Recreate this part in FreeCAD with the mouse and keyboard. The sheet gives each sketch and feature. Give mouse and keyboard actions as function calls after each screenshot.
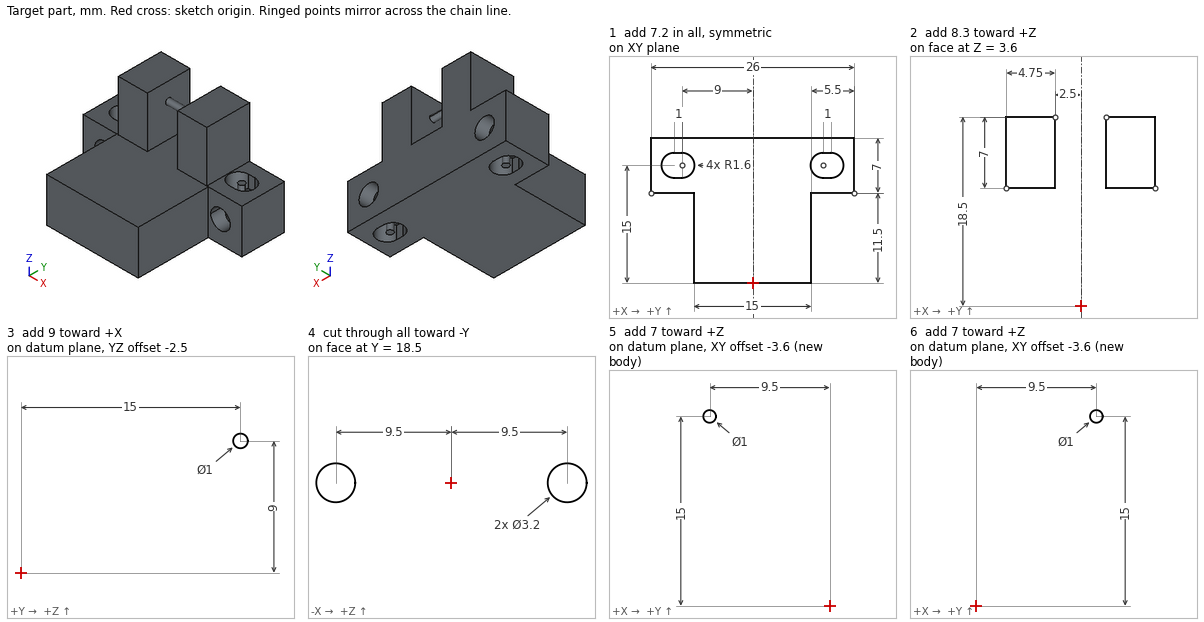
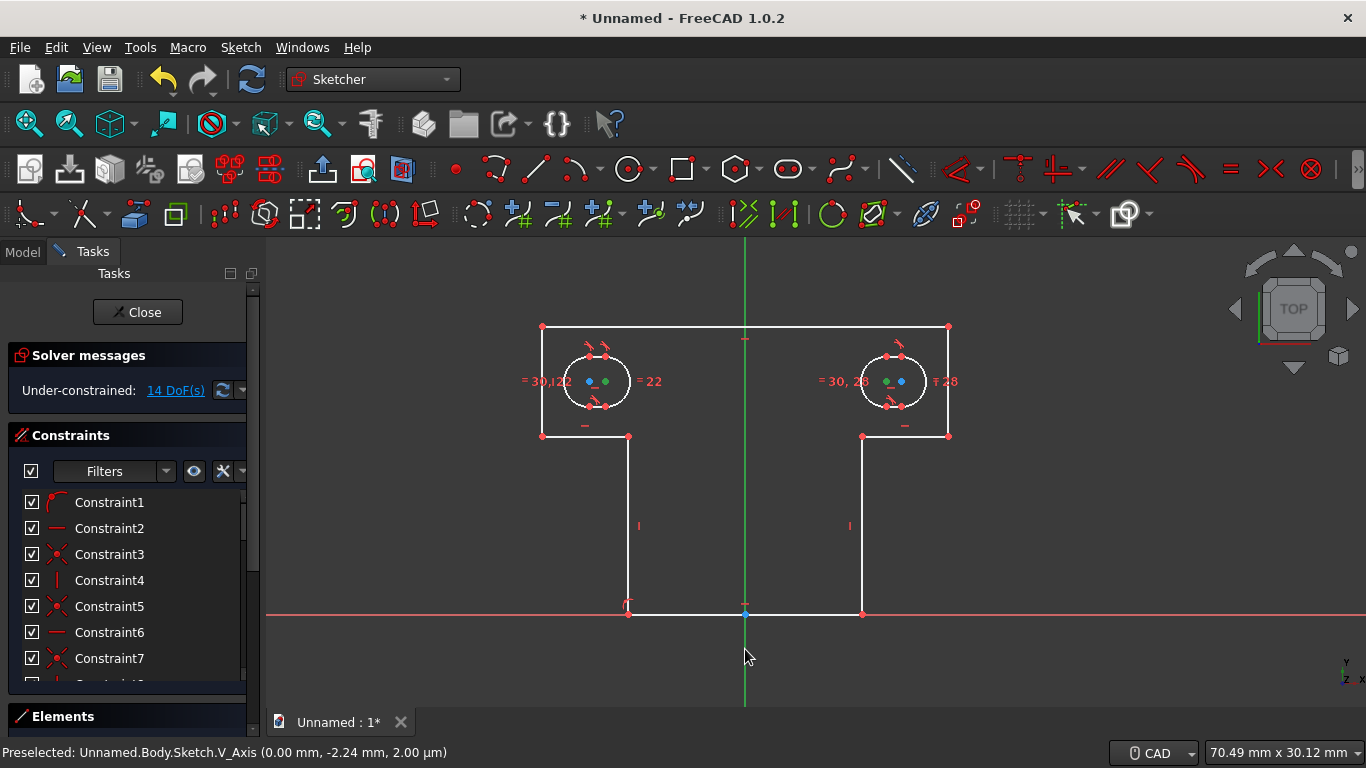
click(1272, 170)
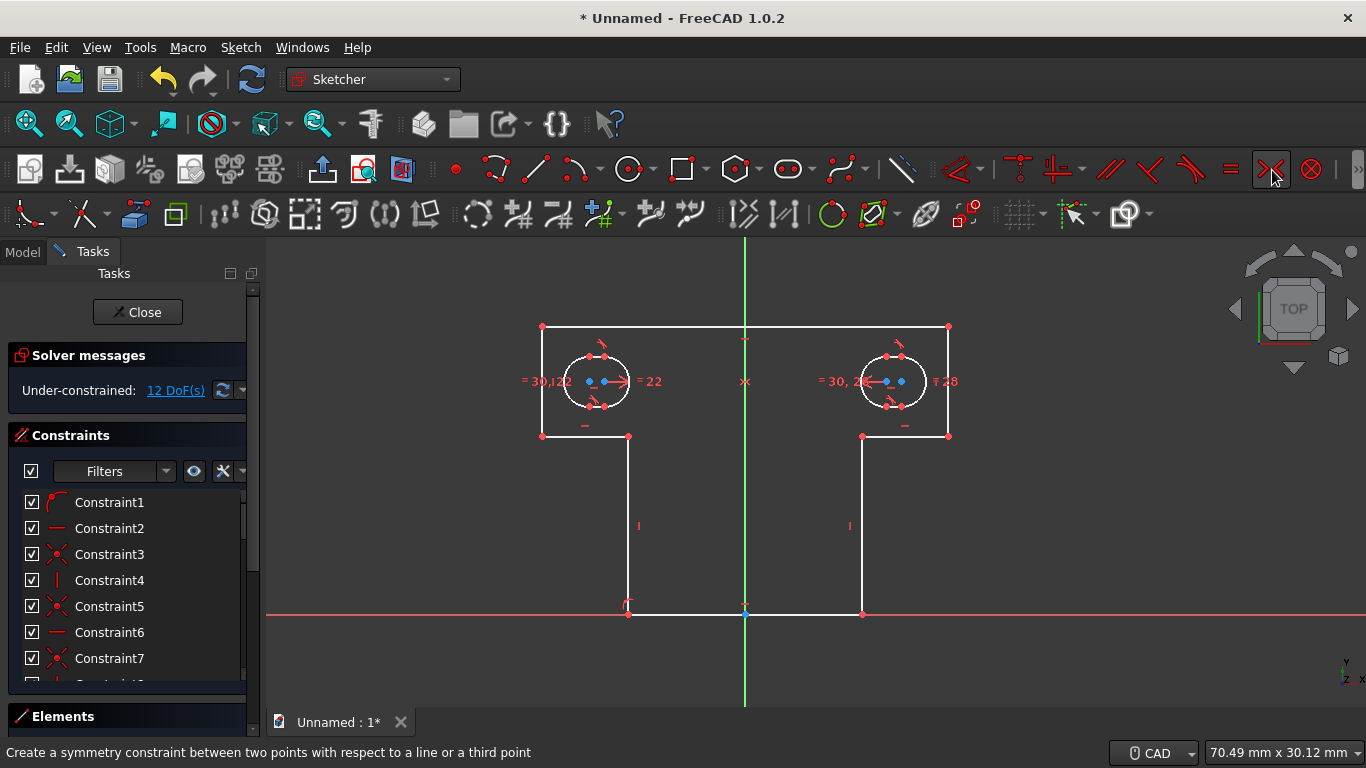
click(948, 437)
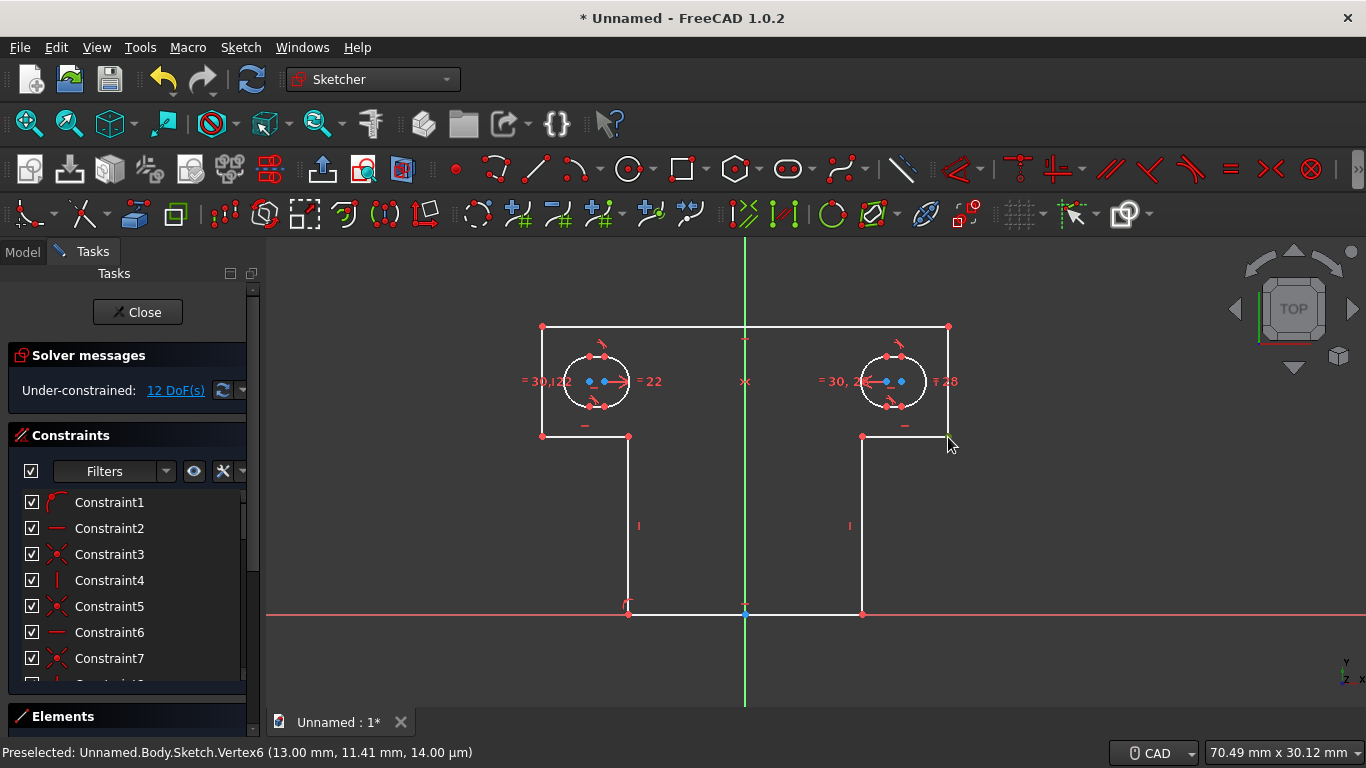
click(542, 437)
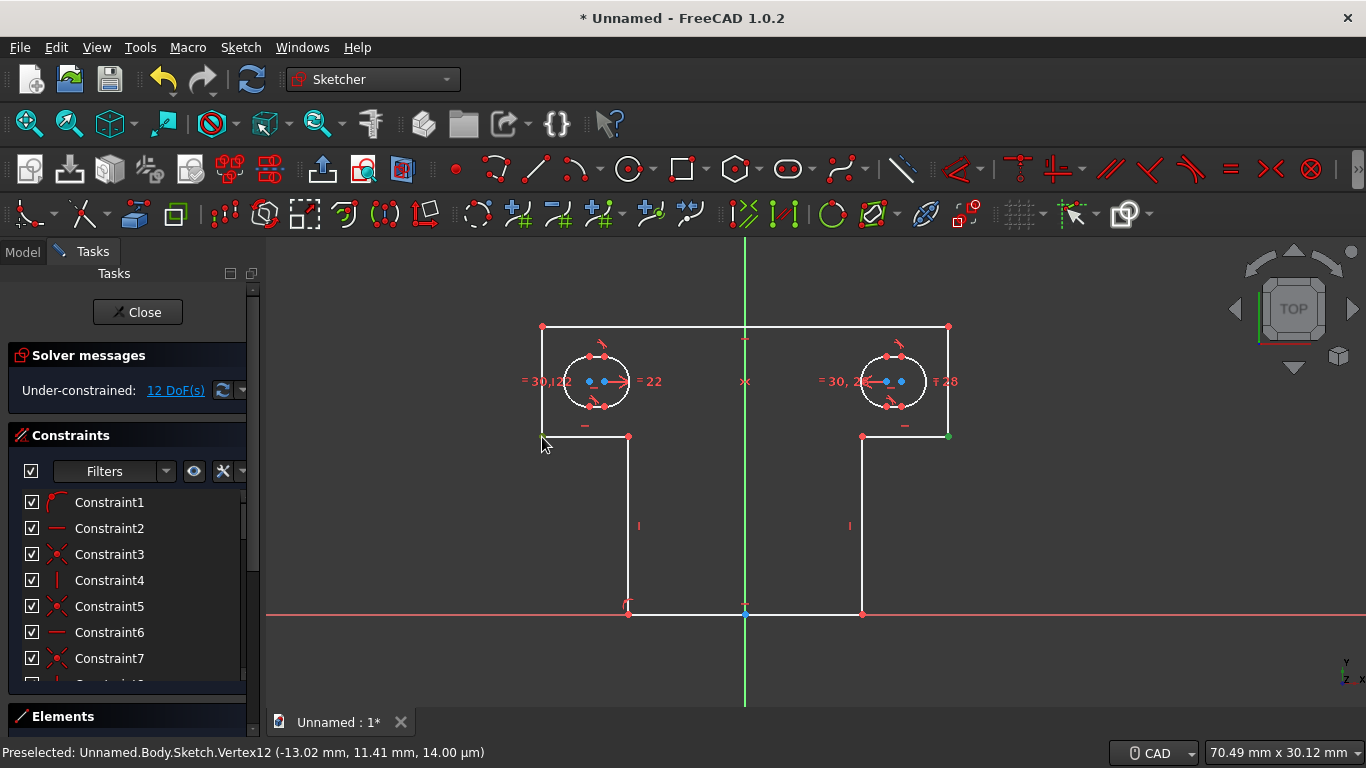
click(745, 649)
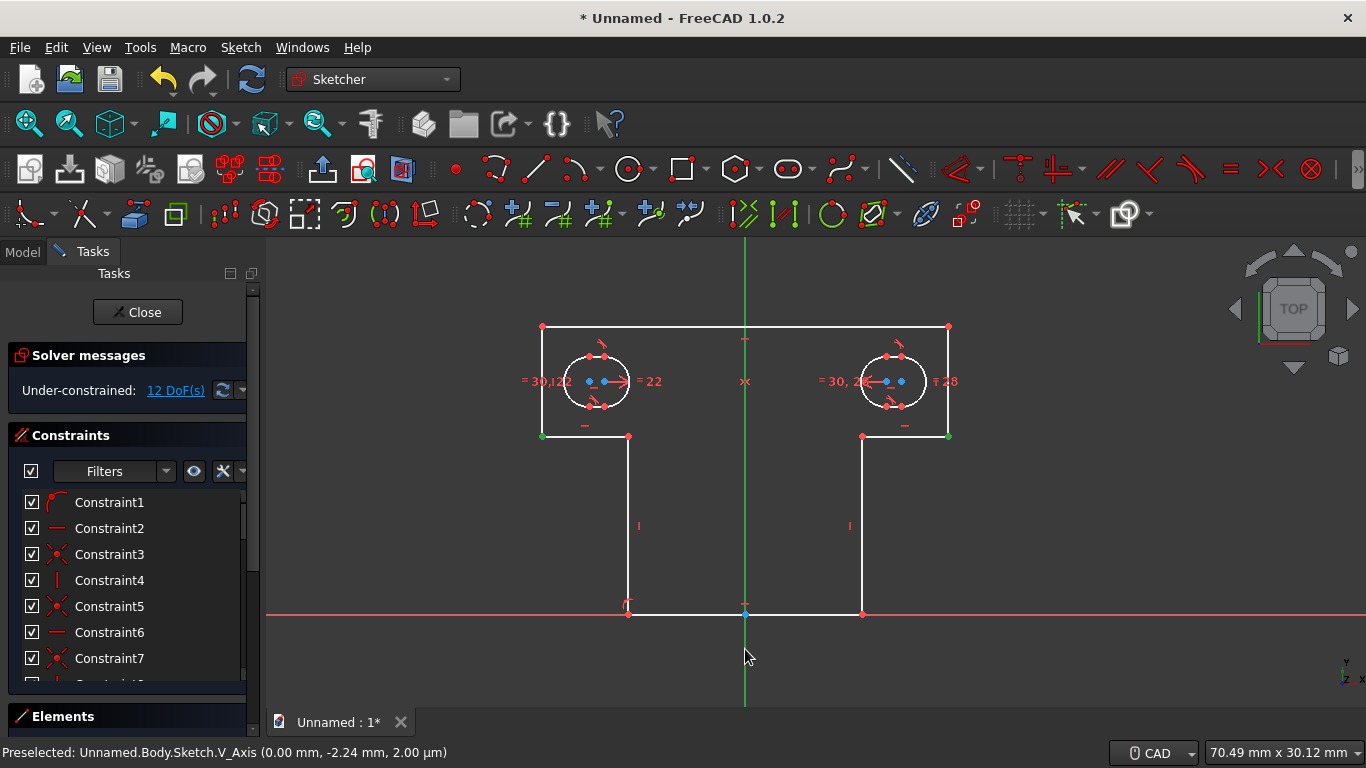
key(s)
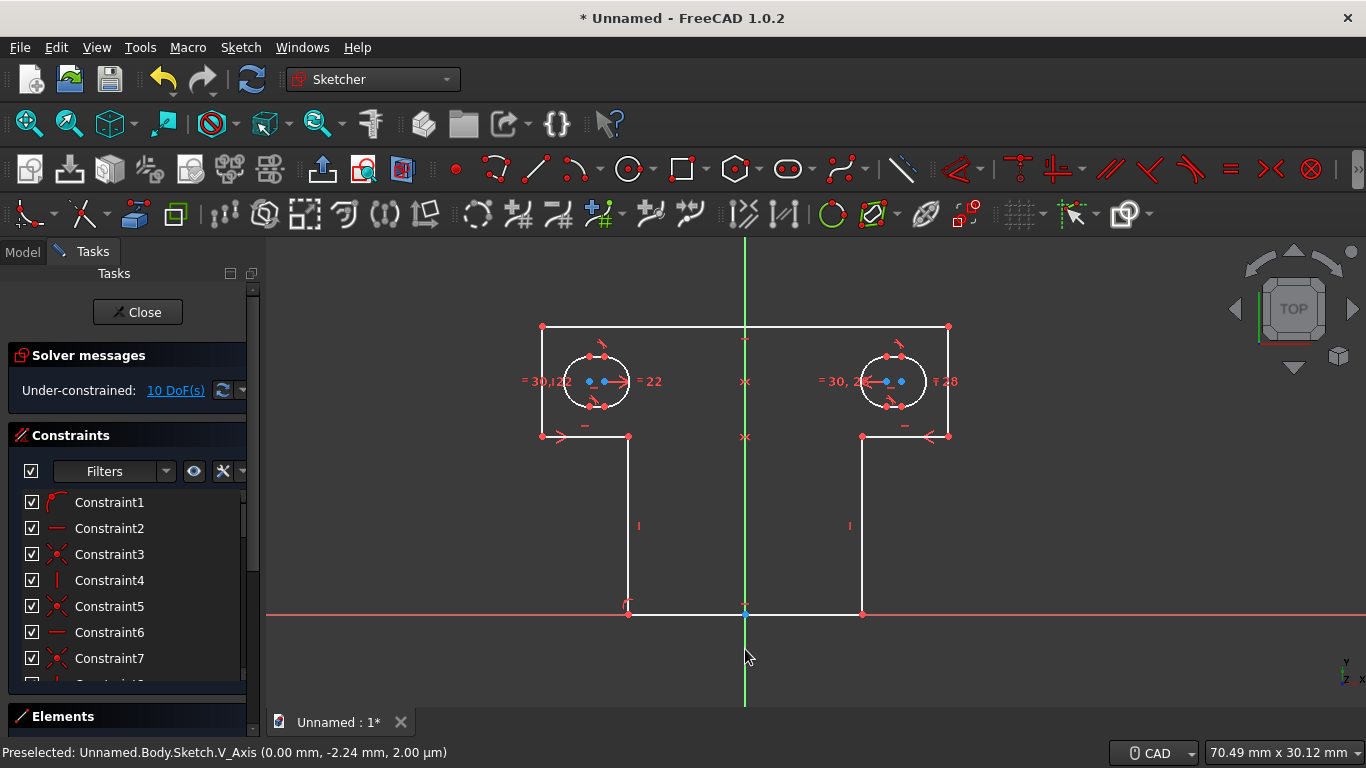
scroll(569, 367, up, 3)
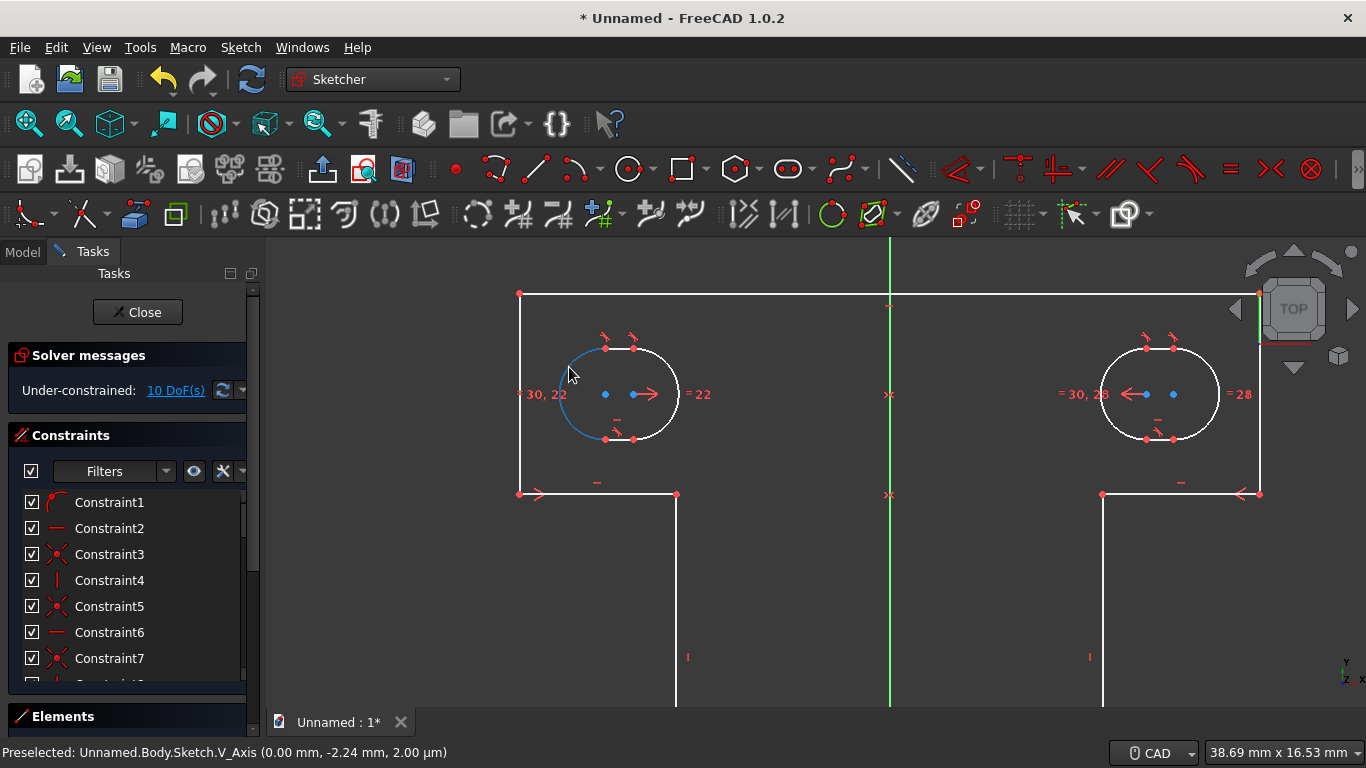
click(568, 367)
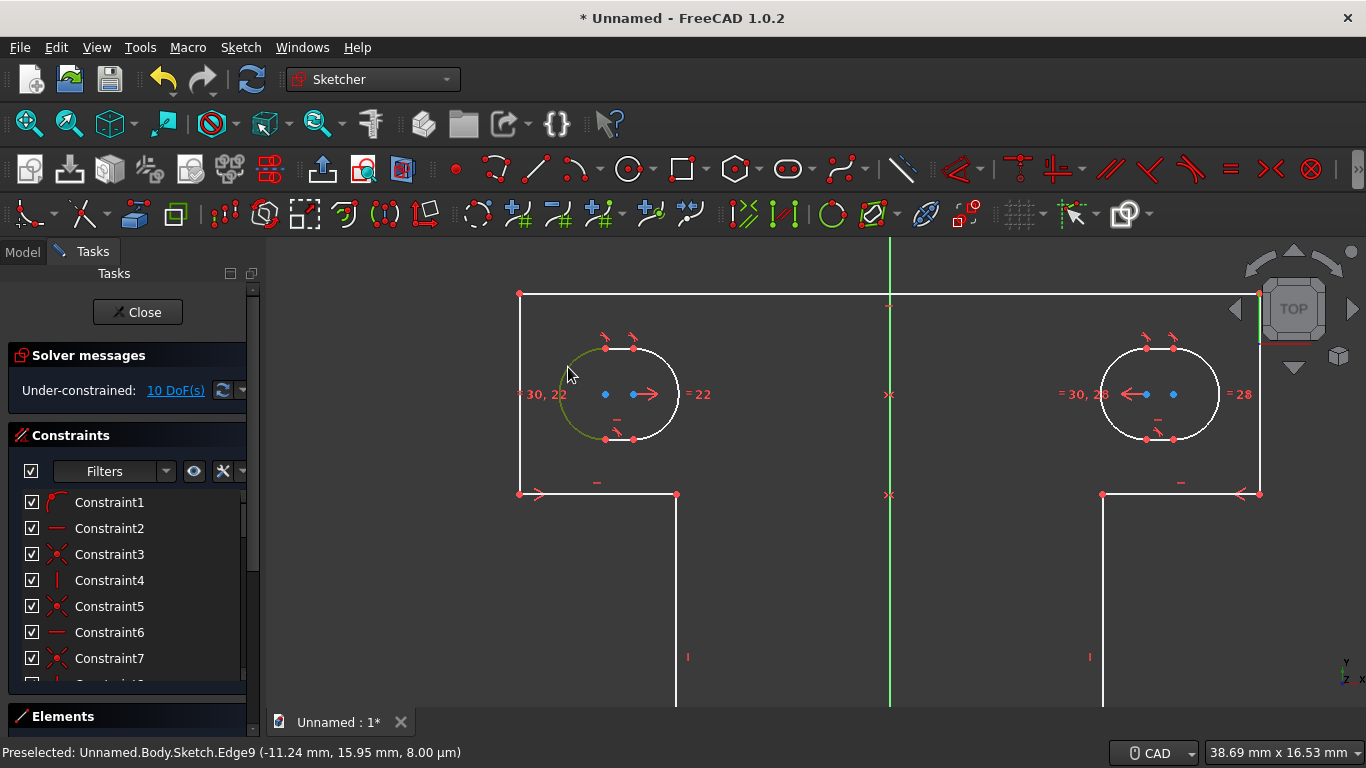
key(k)
key(r)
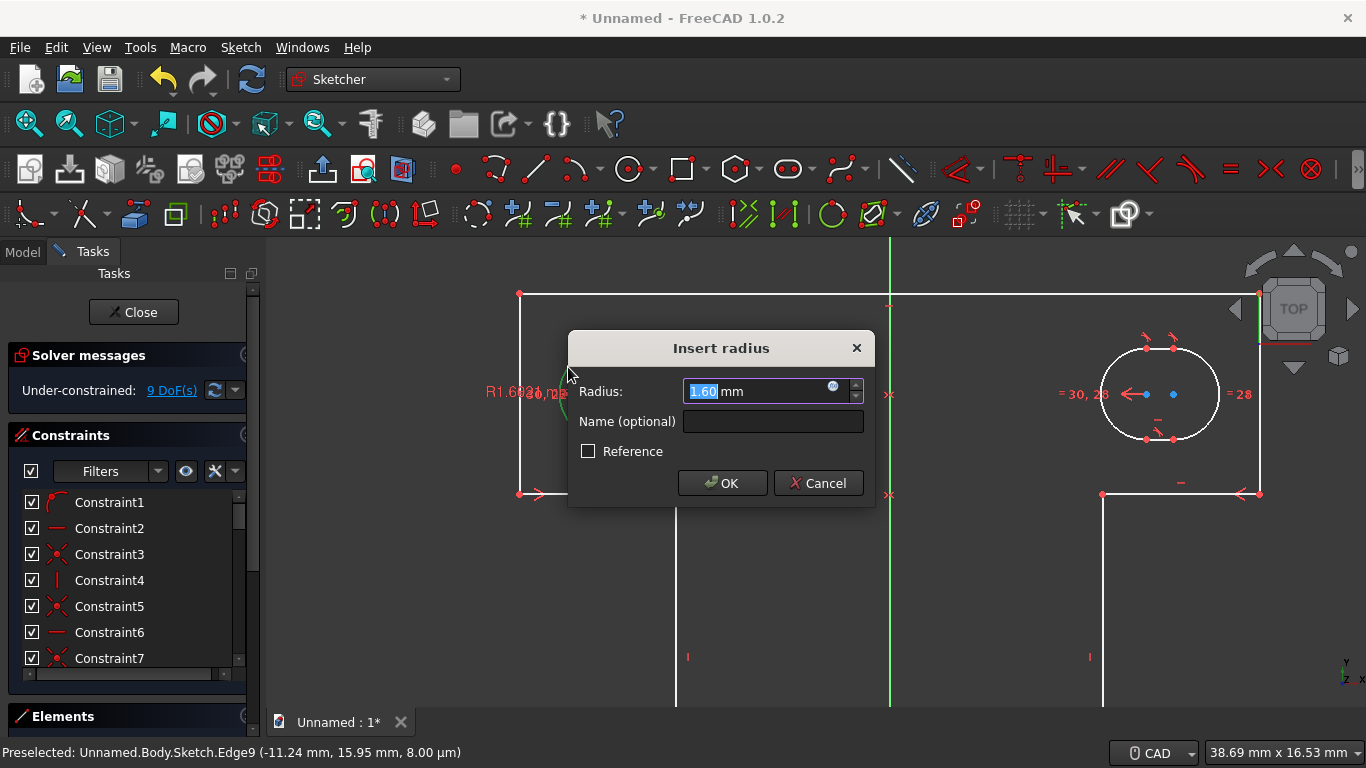
text(1.6)
key(Return)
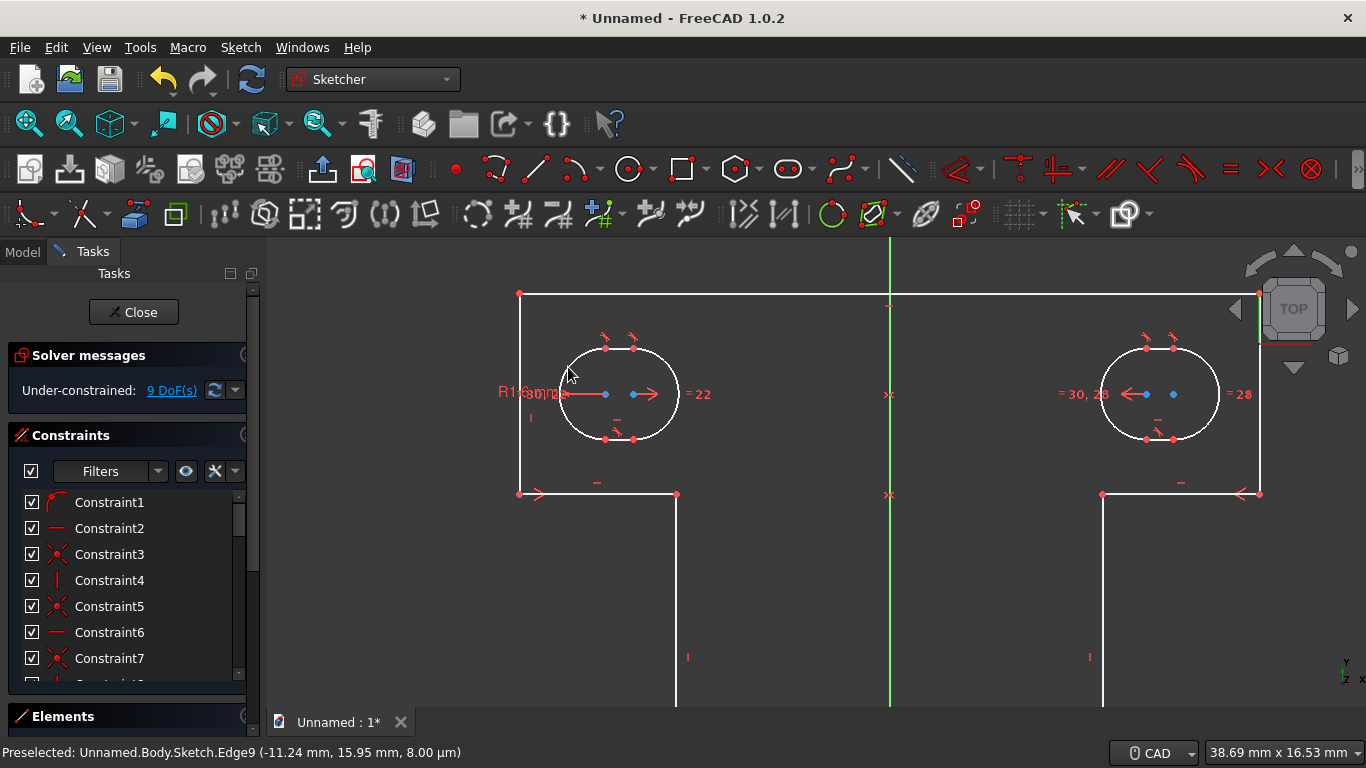
scroll(574, 370, down, 3)